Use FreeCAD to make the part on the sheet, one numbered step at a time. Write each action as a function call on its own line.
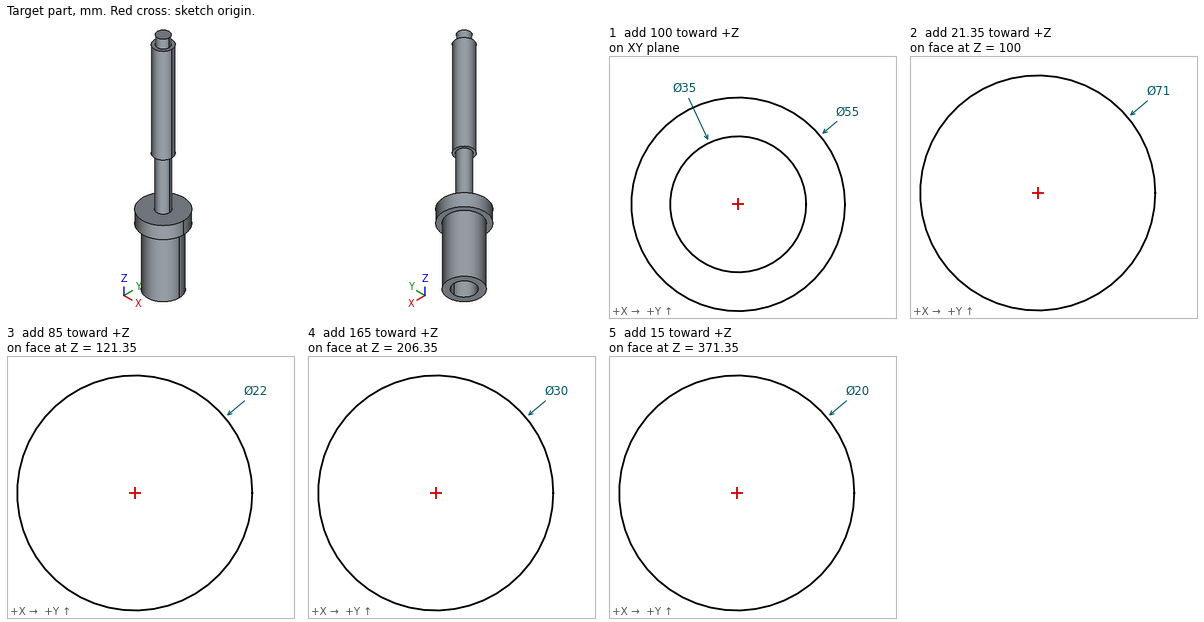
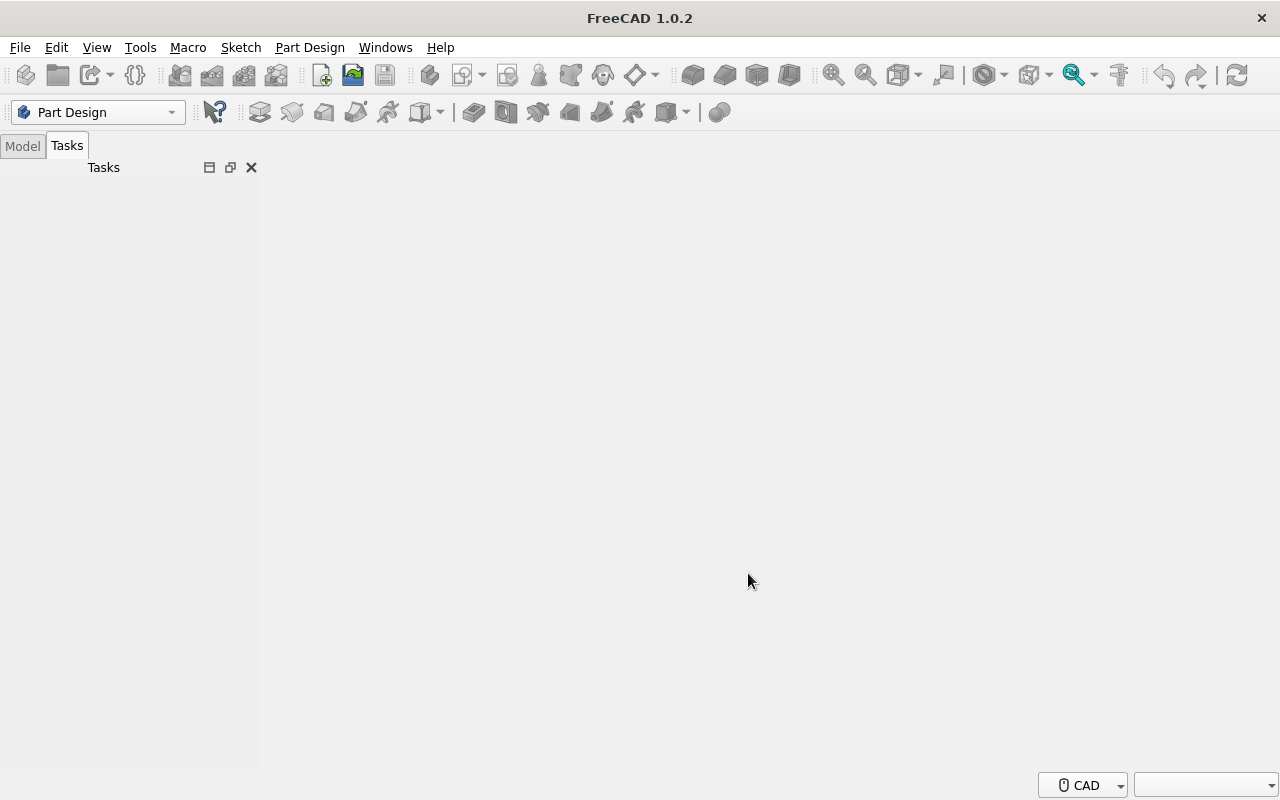
key(ctrl+n)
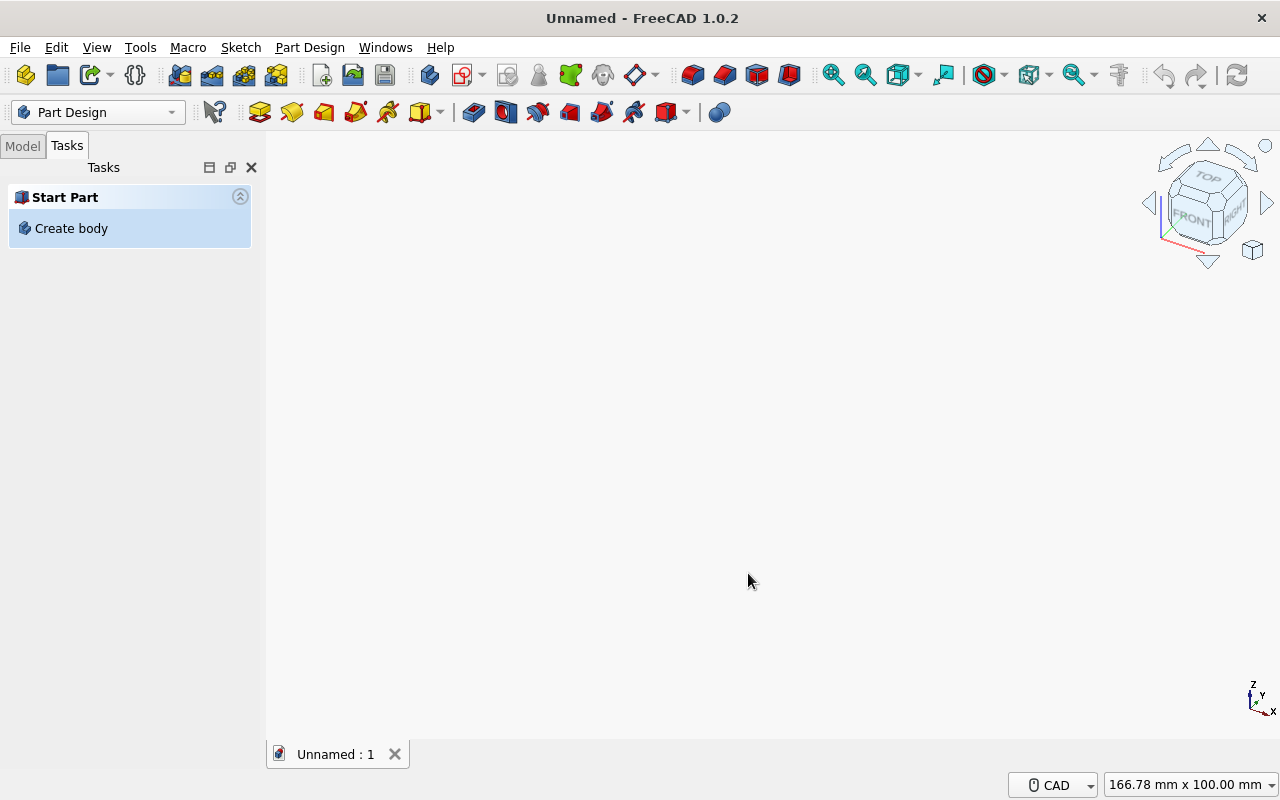
click(462, 76)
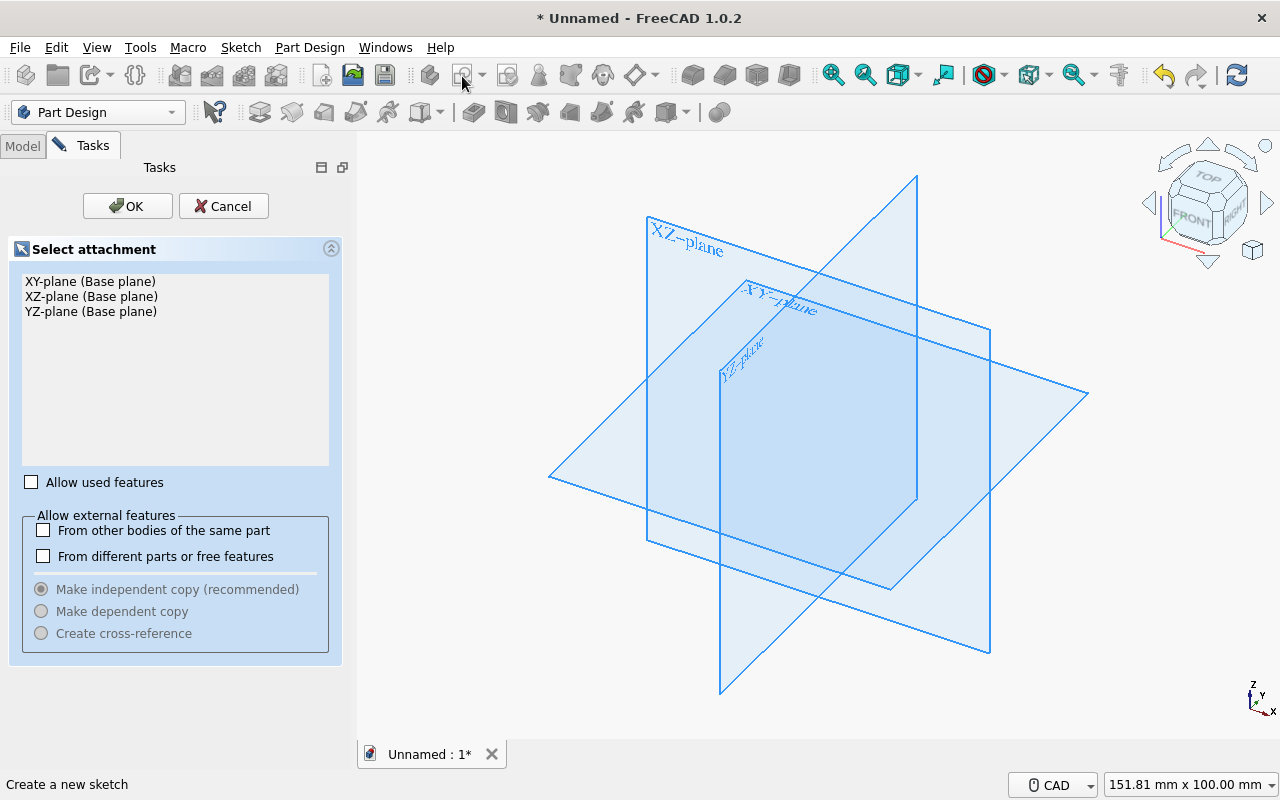
click(82, 282)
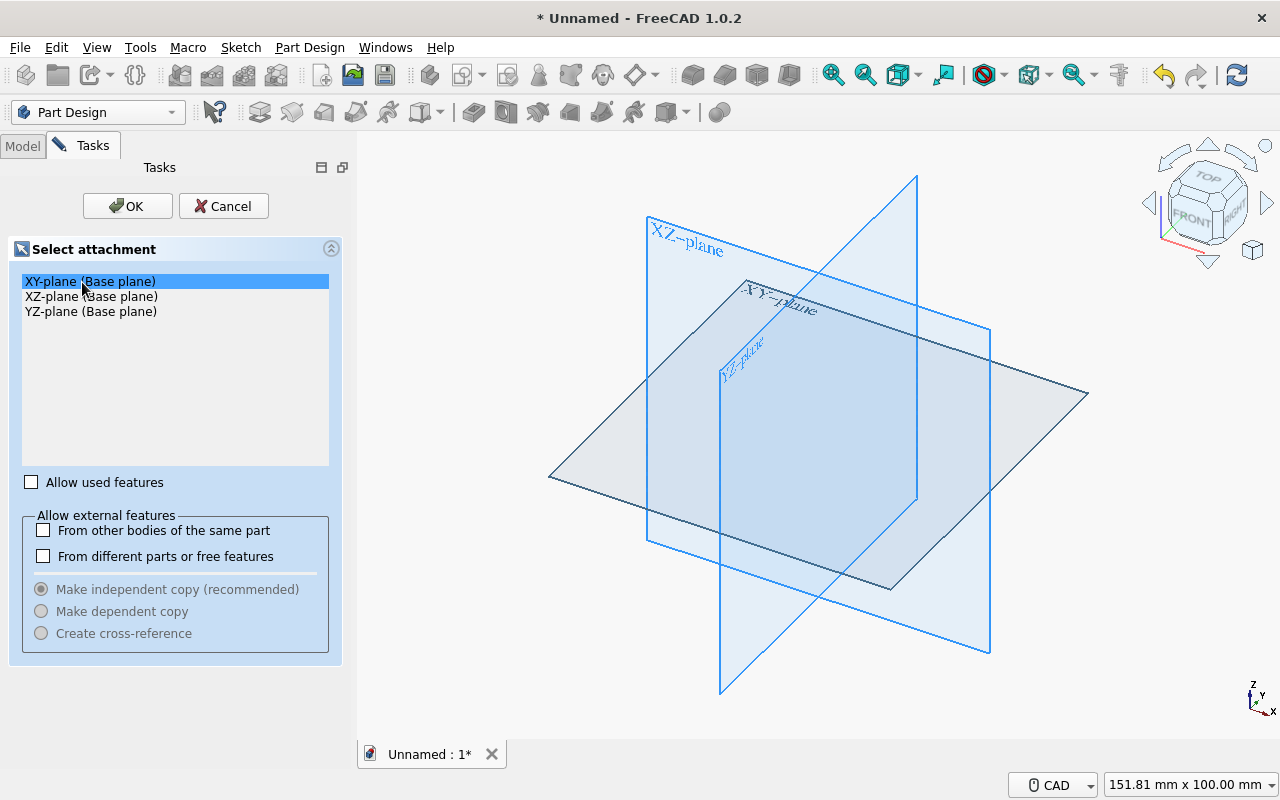
click(128, 206)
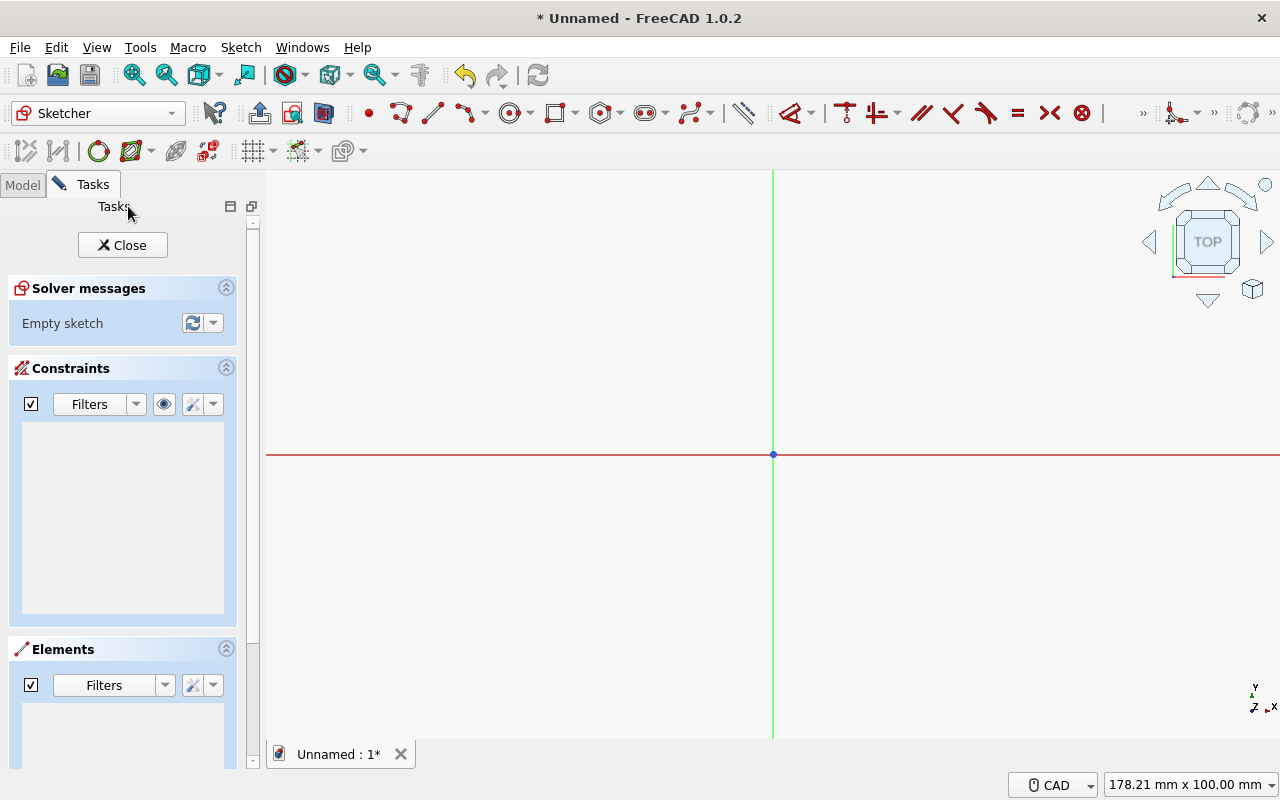
key(g)
key(c)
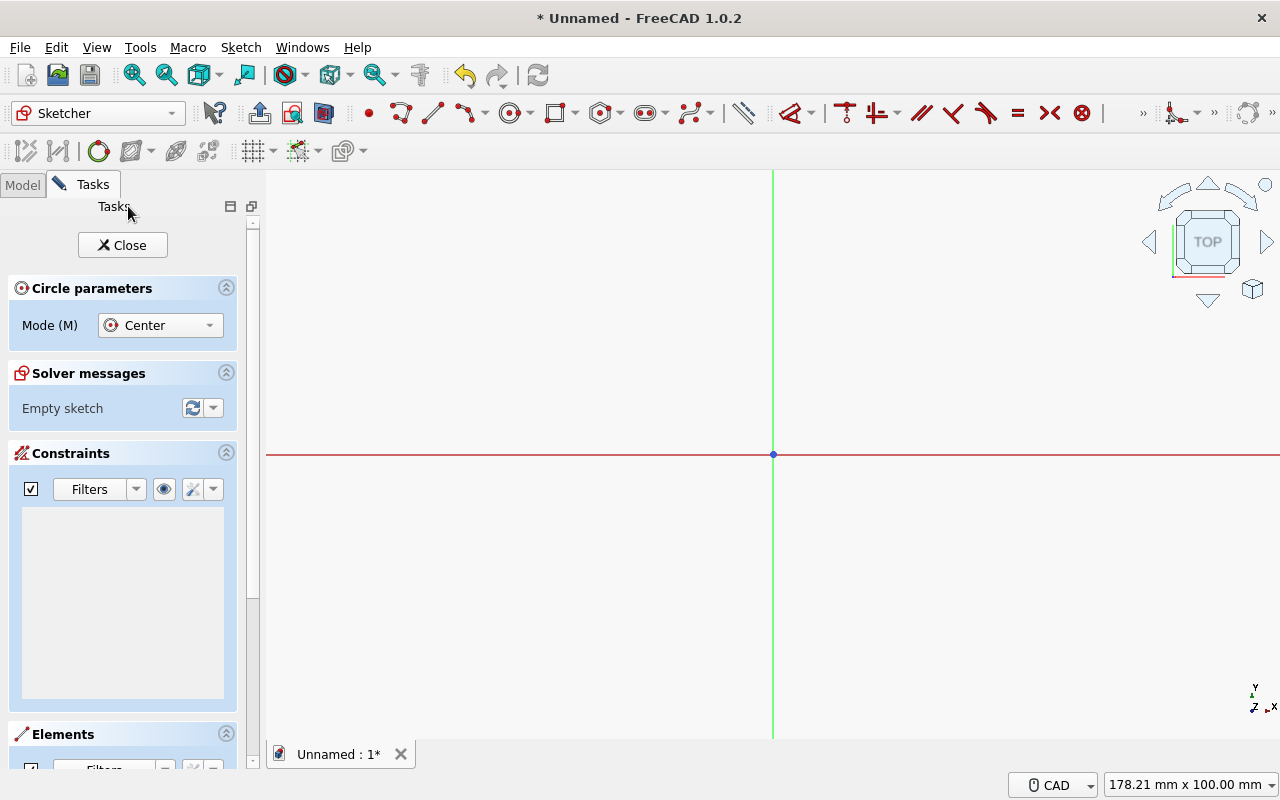
click(773, 454)
click(884, 344)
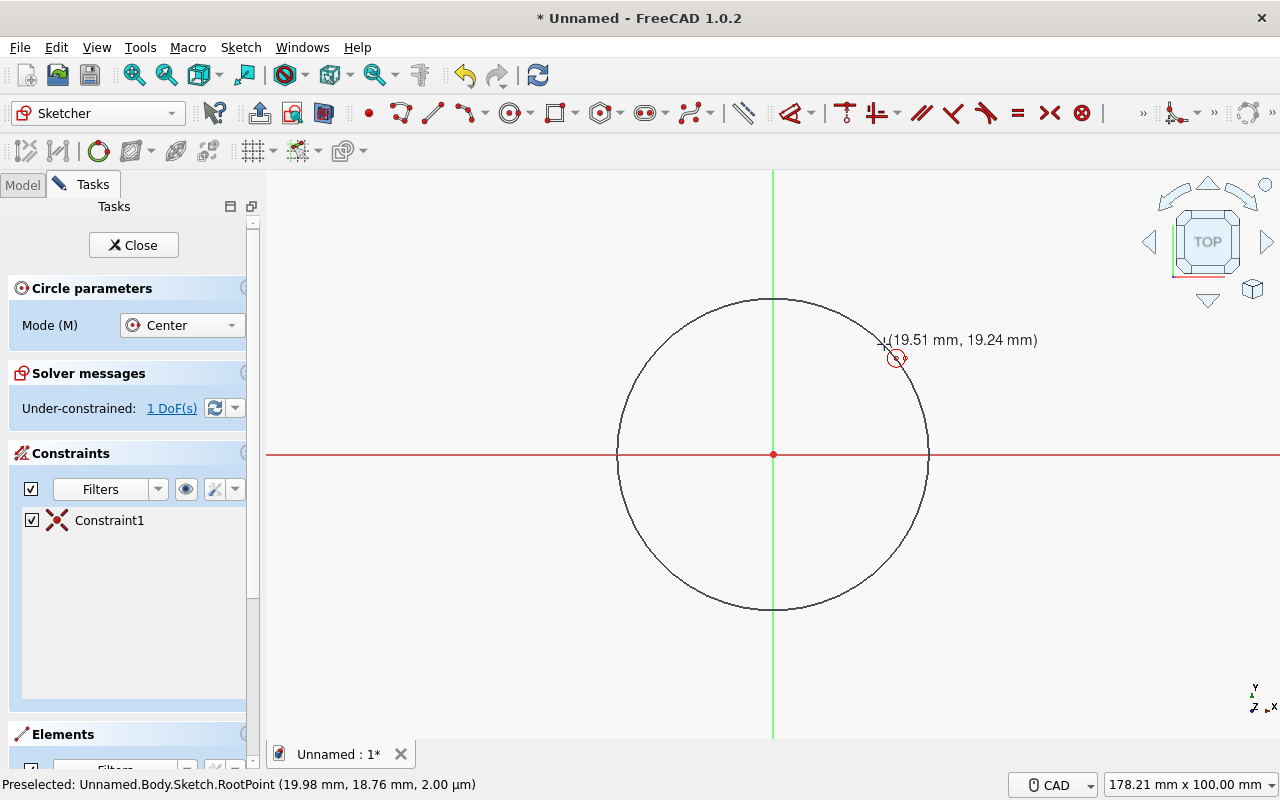
click(773, 454)
click(843, 384)
key(Escape)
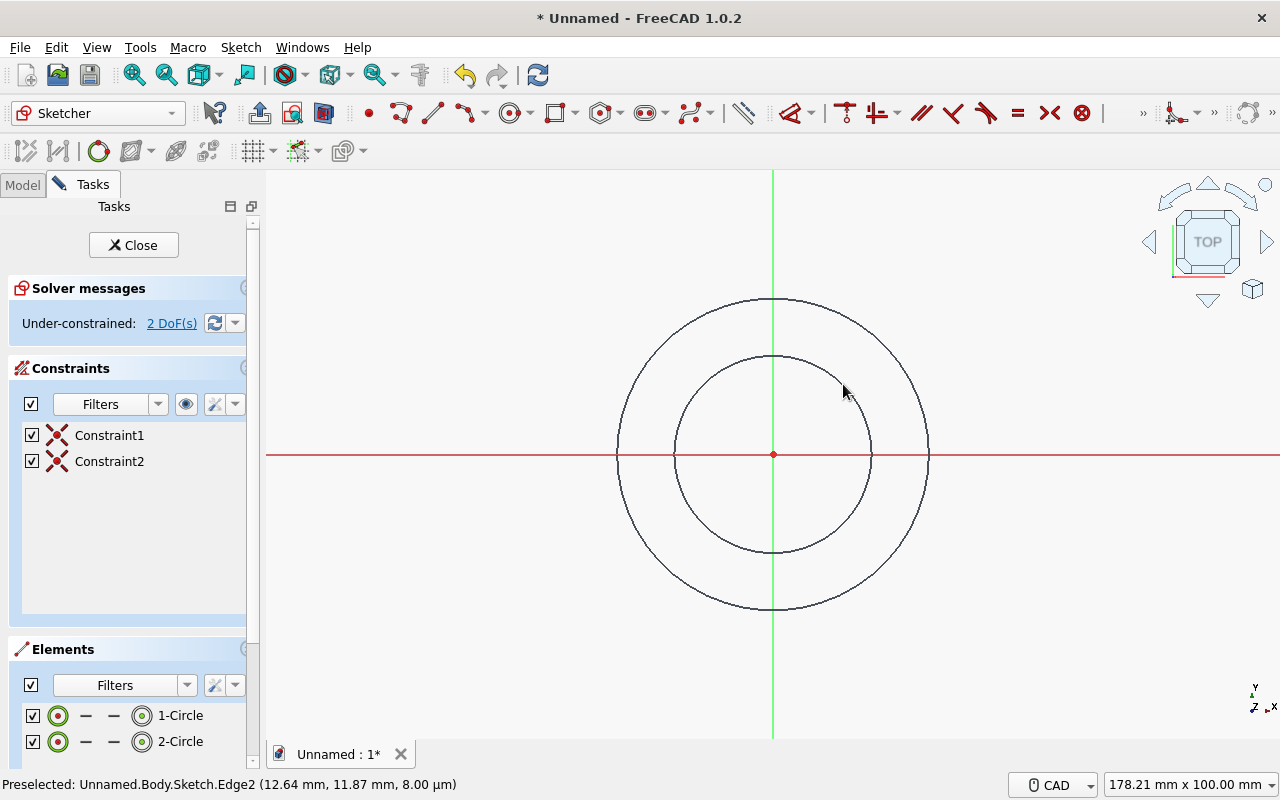
click(883, 344)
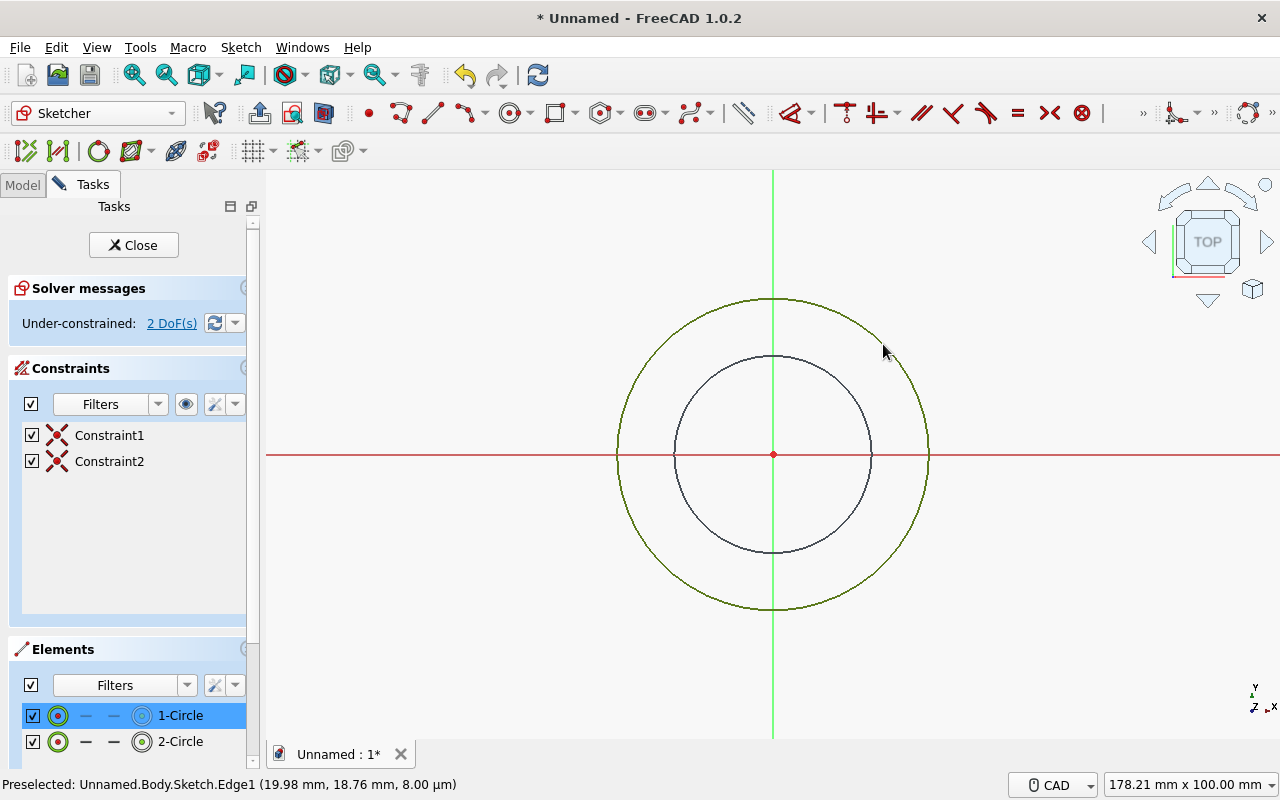
key(k)
key(o)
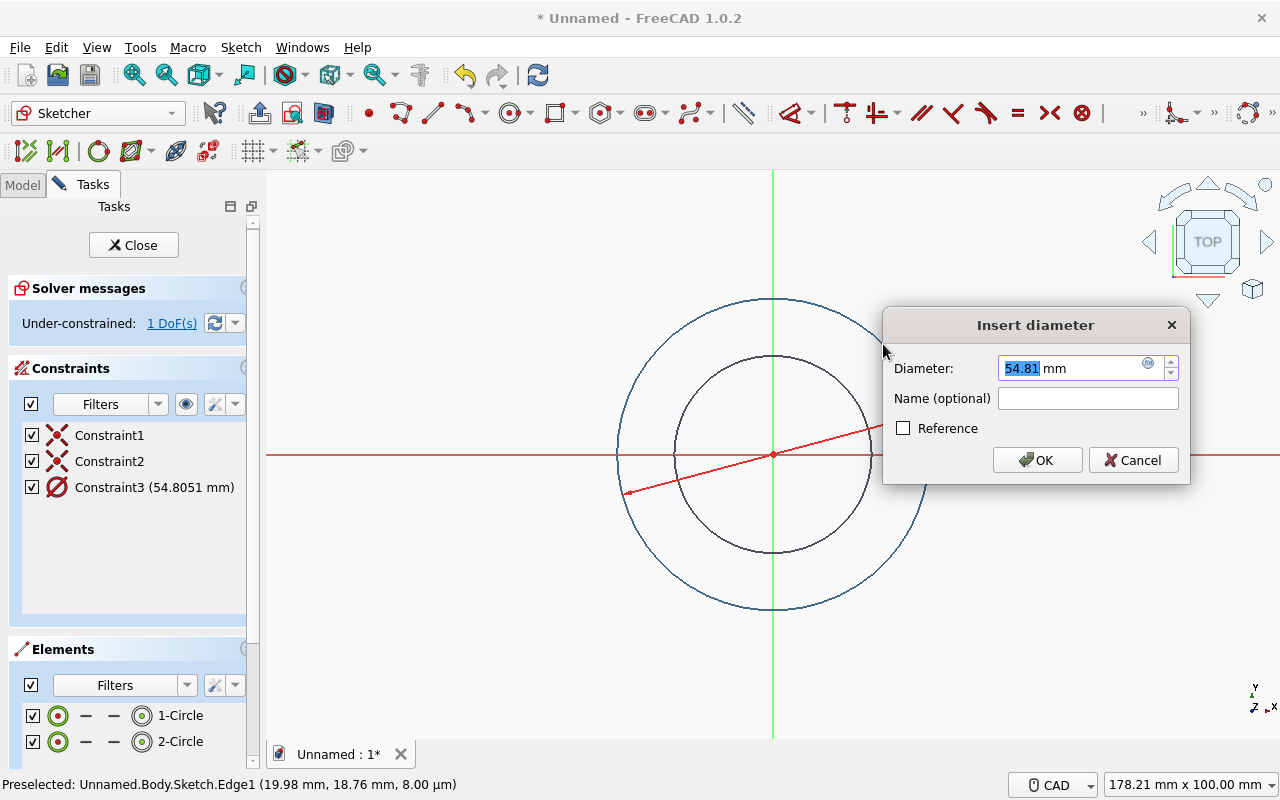
text(55)
key(Return)